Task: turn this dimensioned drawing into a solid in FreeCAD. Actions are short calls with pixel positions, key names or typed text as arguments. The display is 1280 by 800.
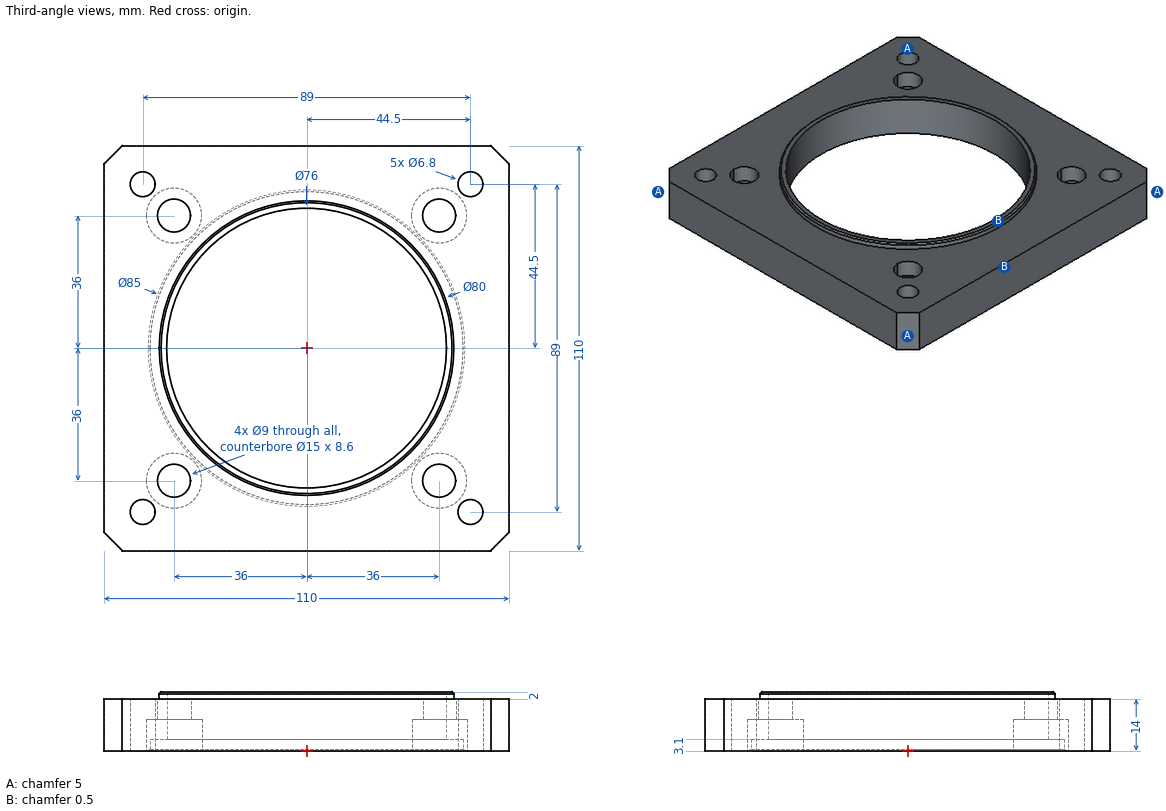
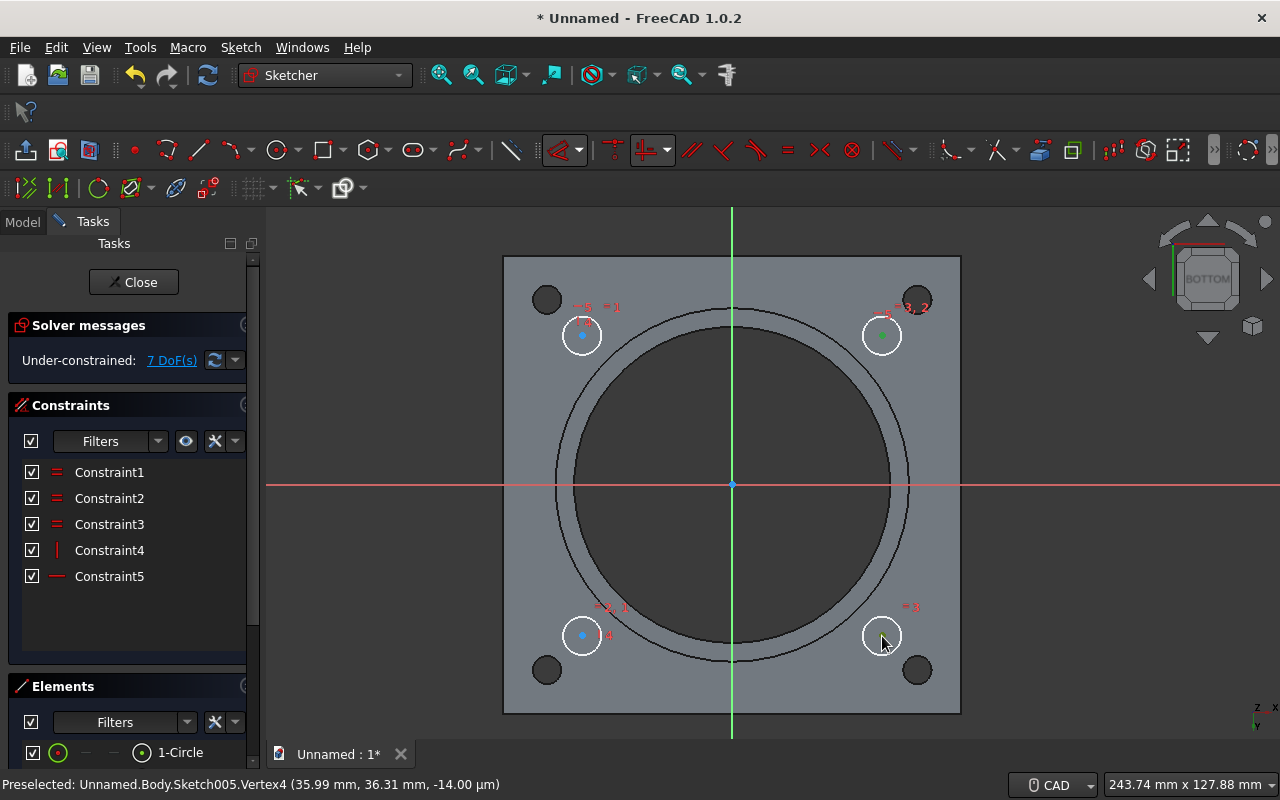
click(670, 150)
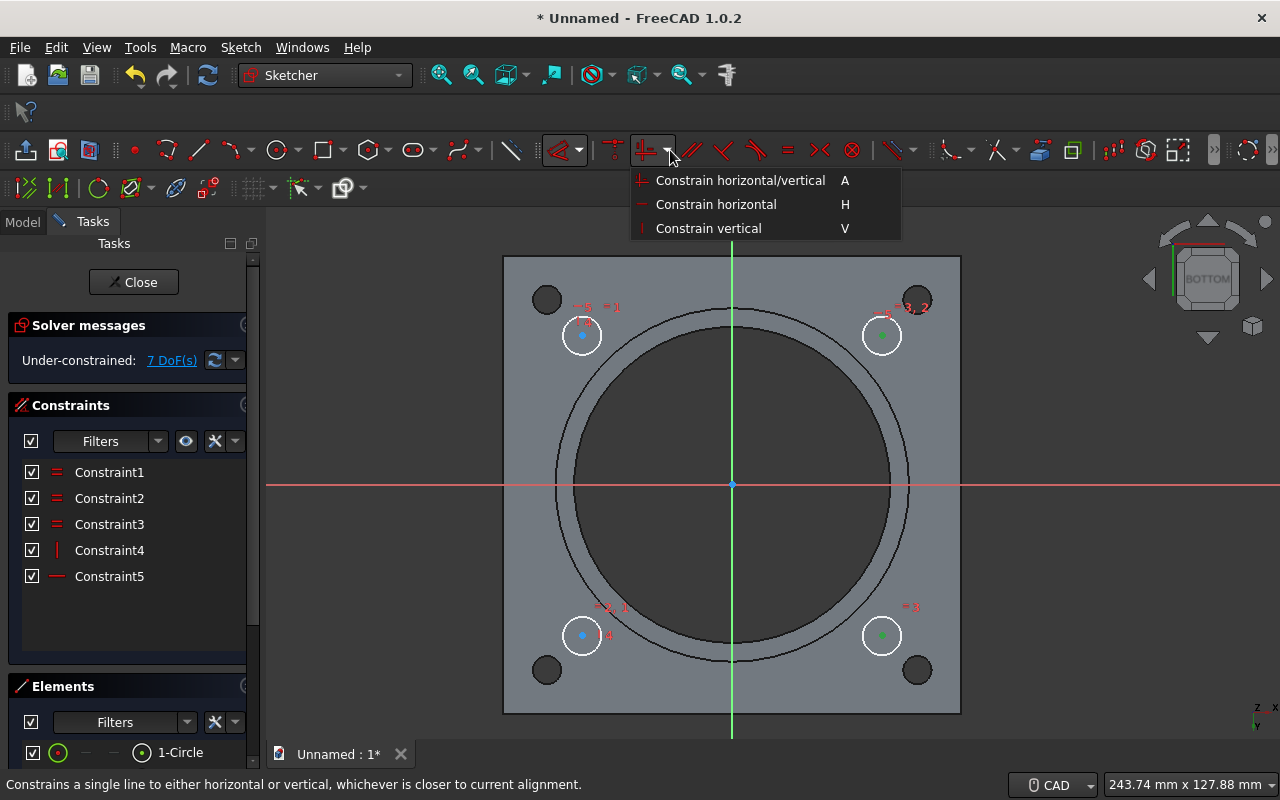
click(766, 228)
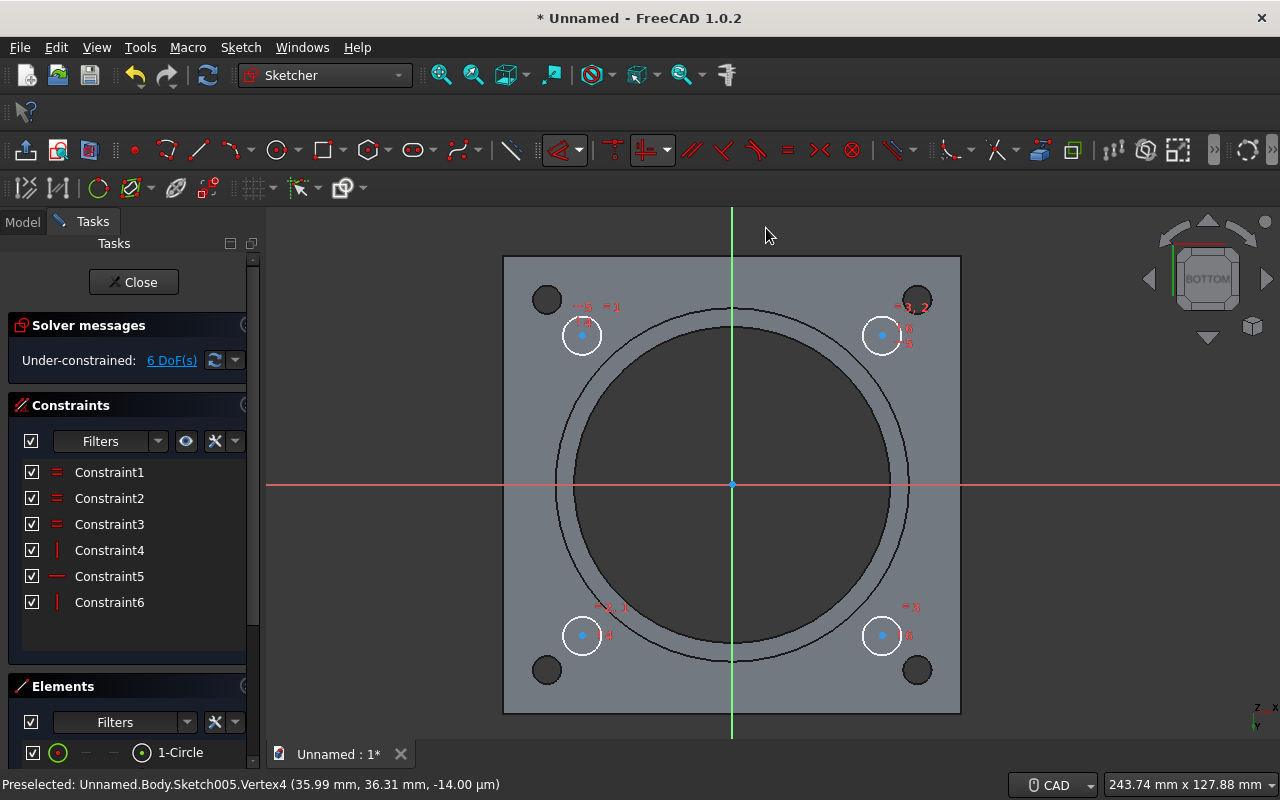
click(582, 636)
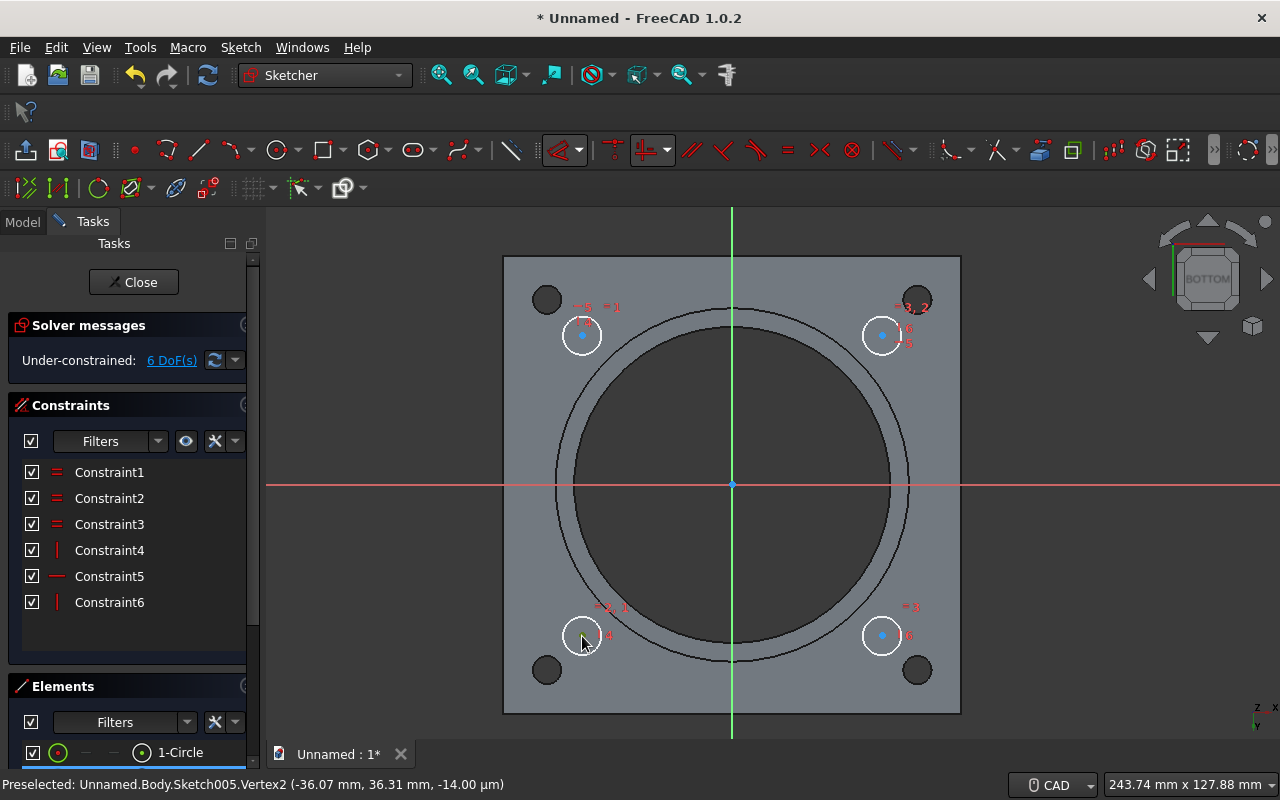
click(882, 636)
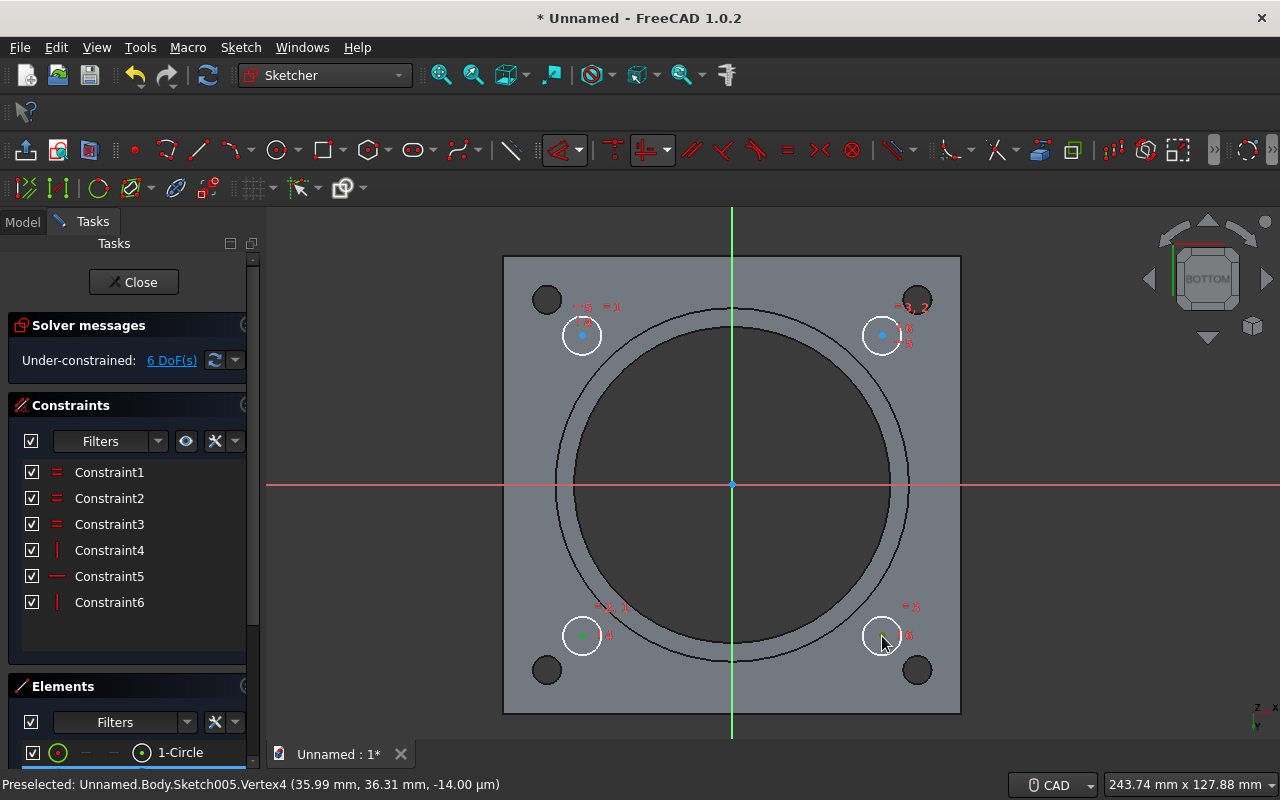
key(h)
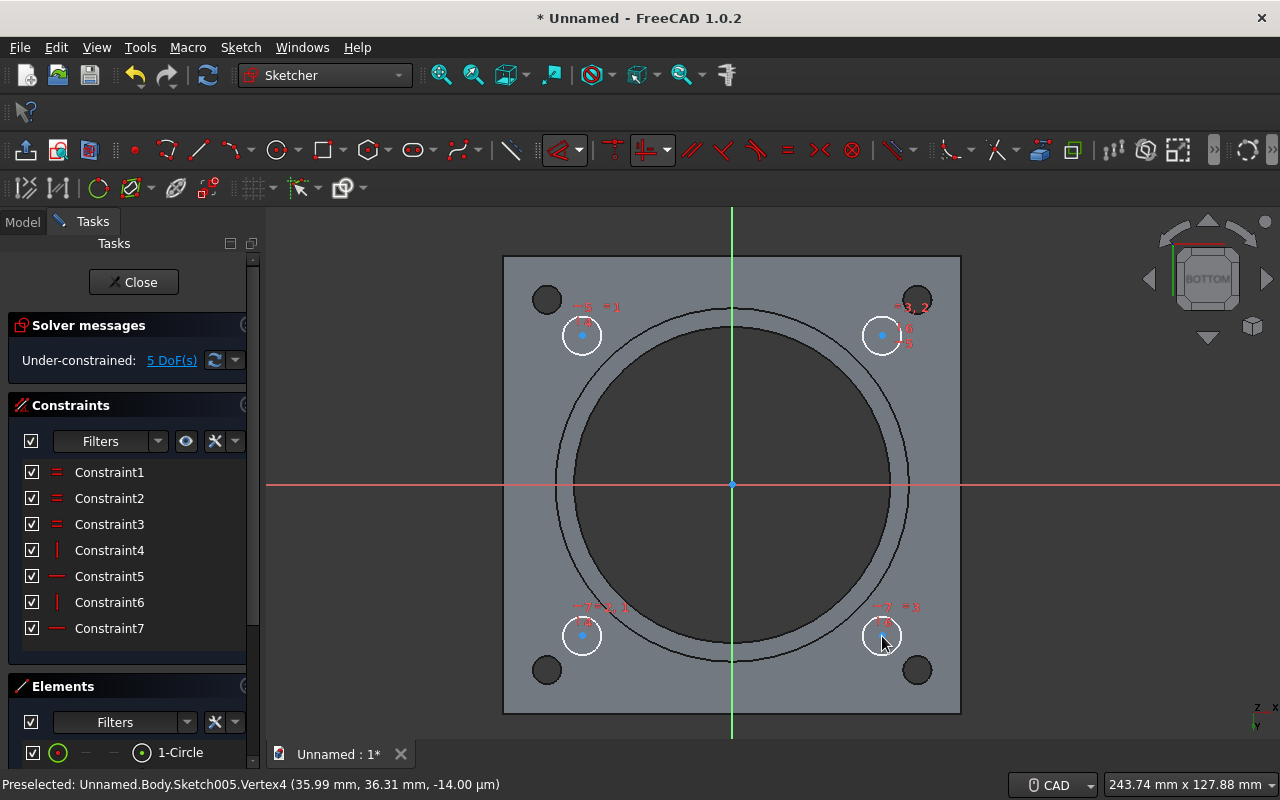
click(596, 322)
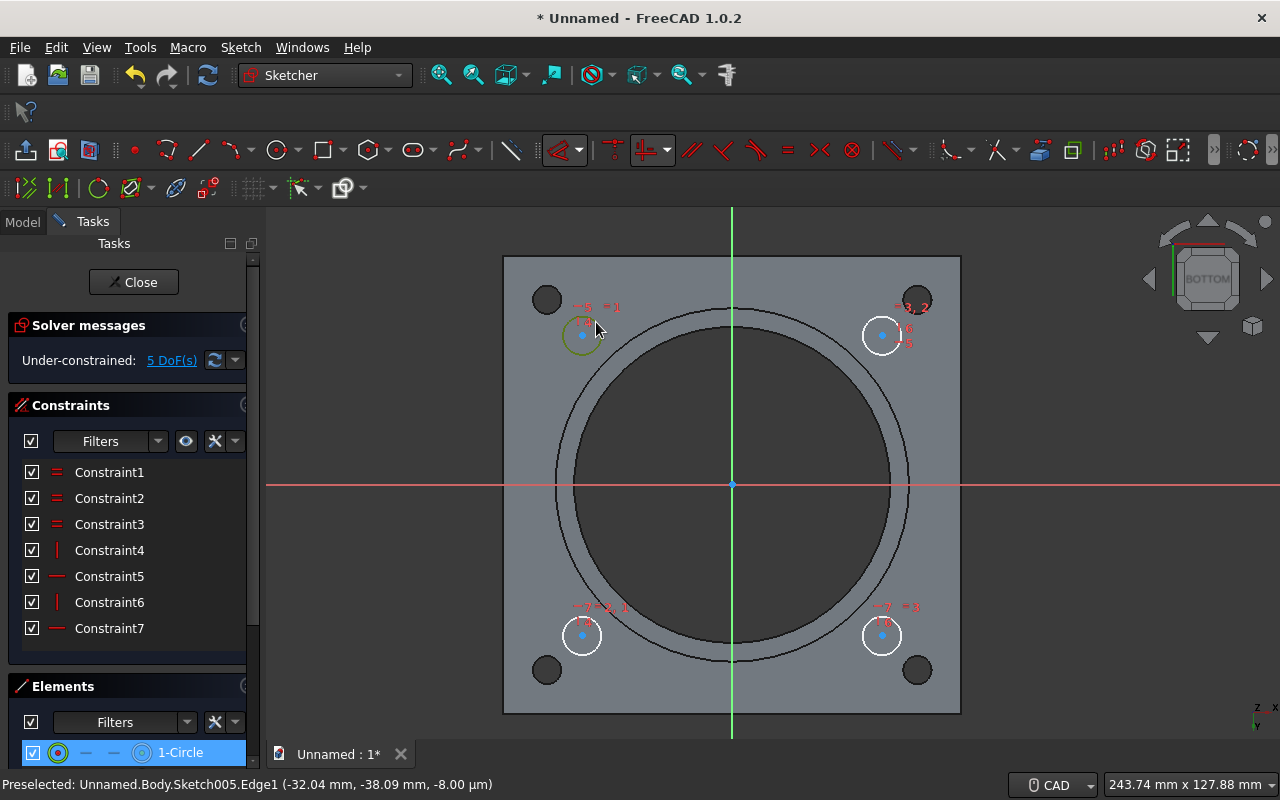
click(582, 150)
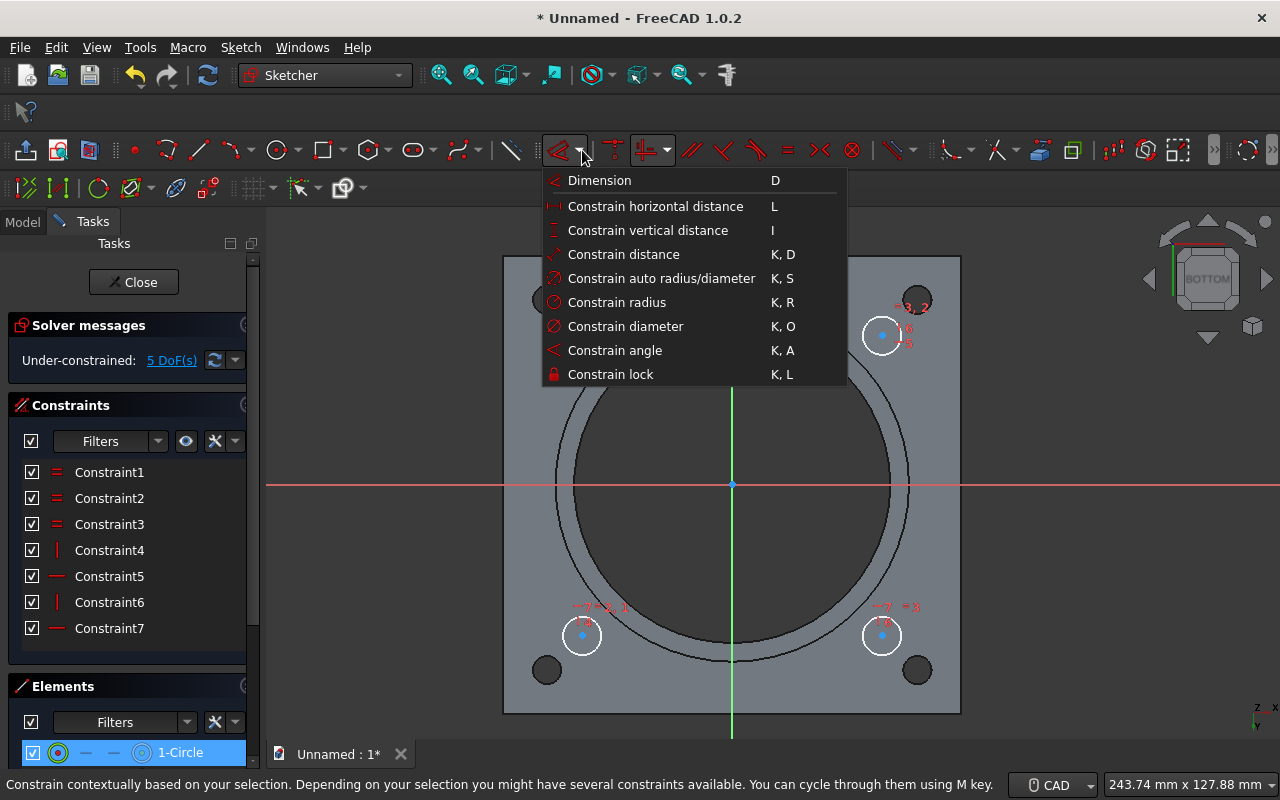
click(695, 326)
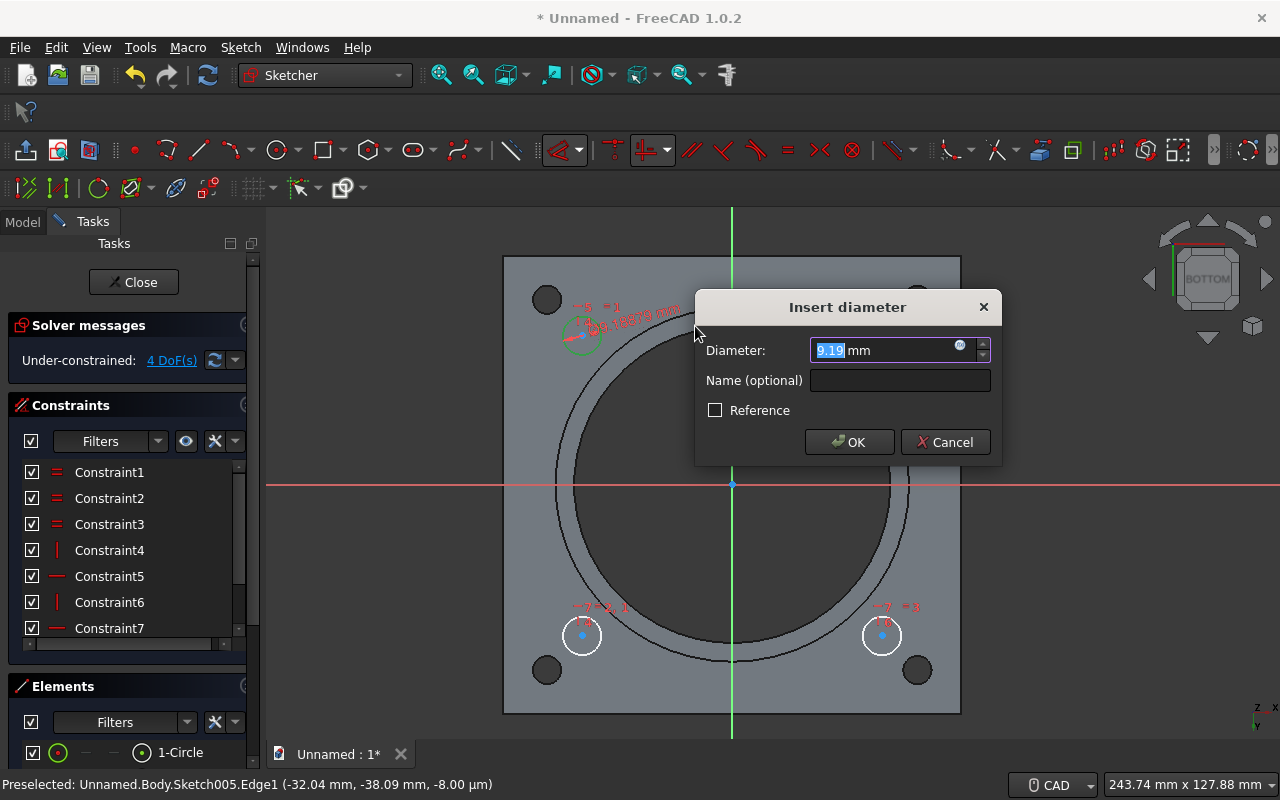
text(9)
key(Return)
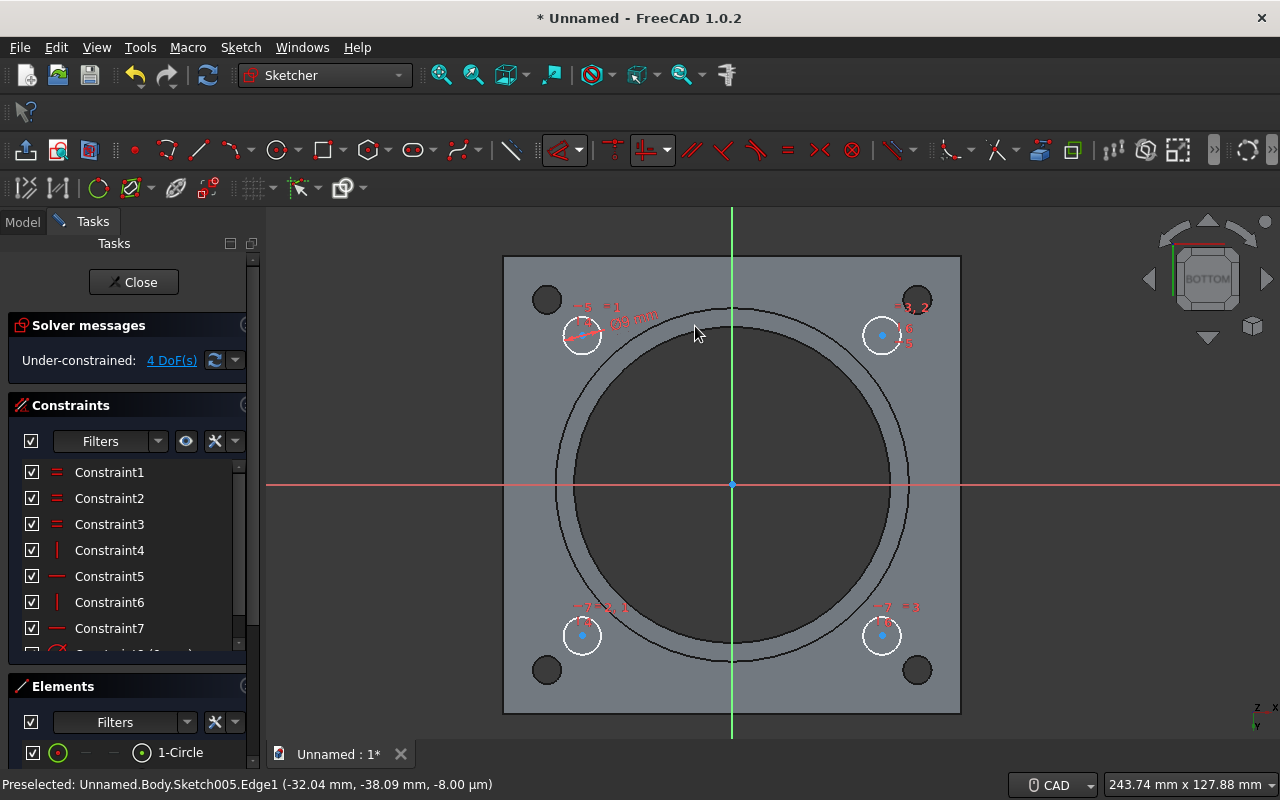
click(582, 336)